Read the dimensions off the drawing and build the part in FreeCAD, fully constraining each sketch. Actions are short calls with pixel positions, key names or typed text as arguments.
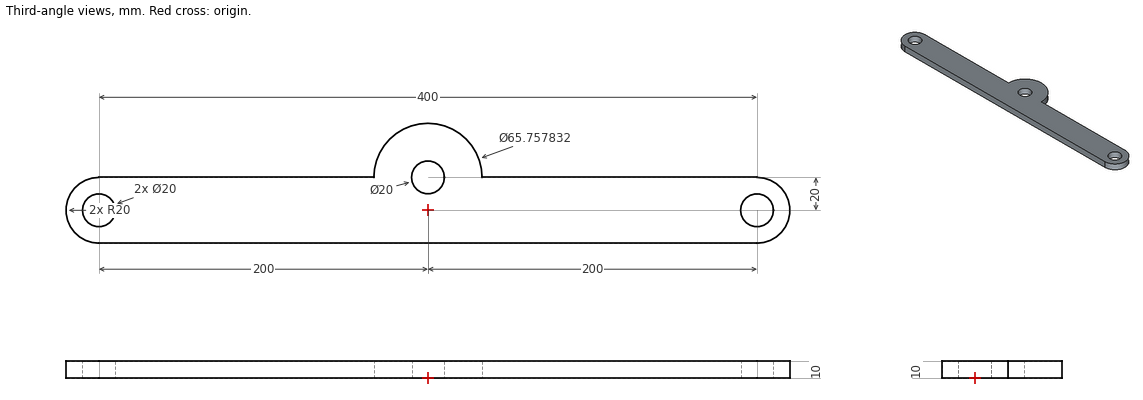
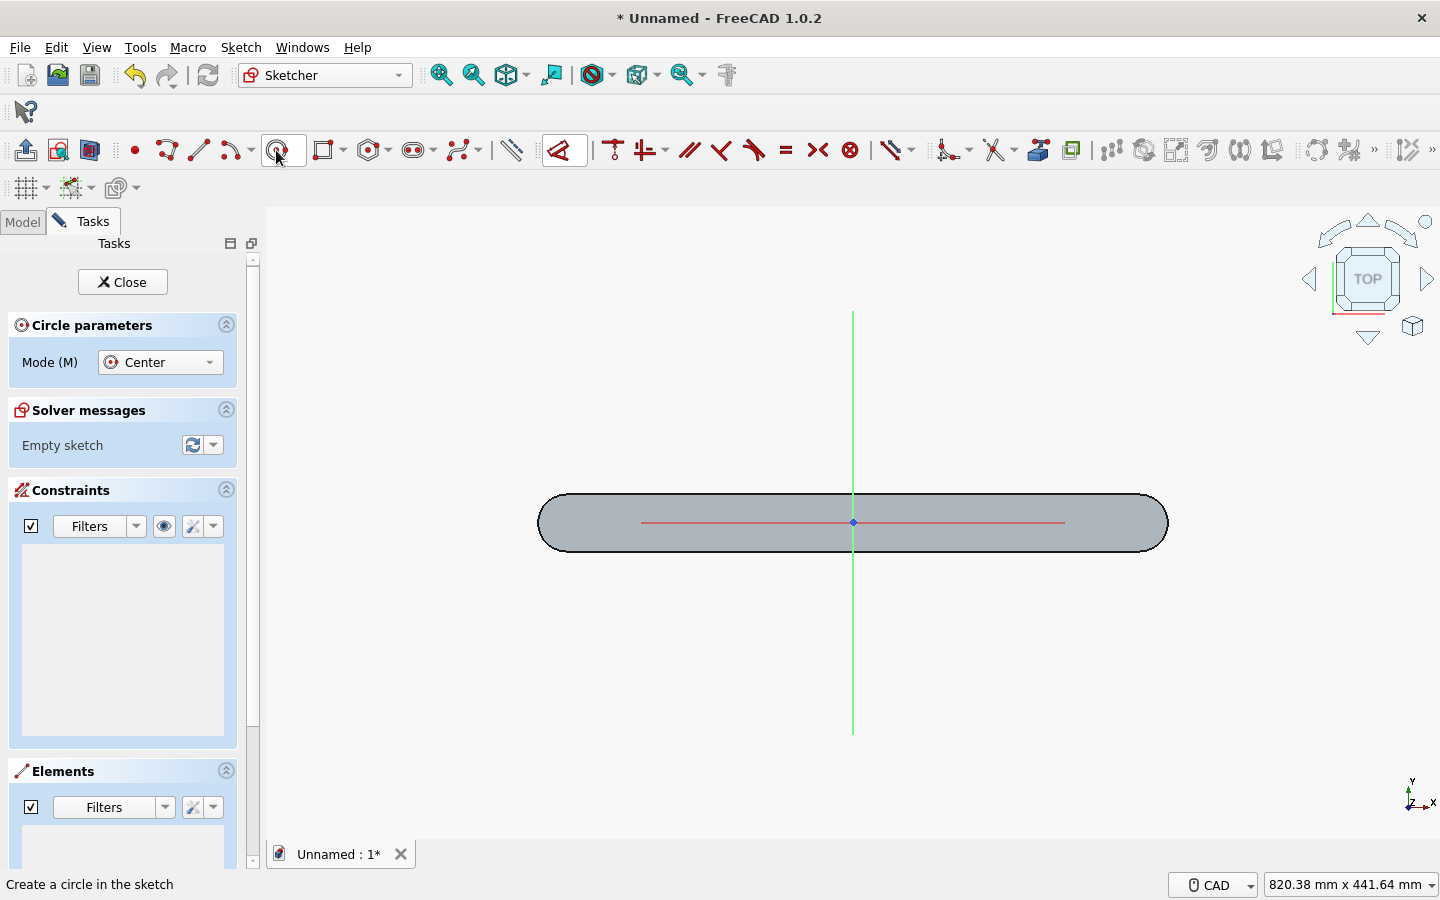
scroll(567, 523, up, 3)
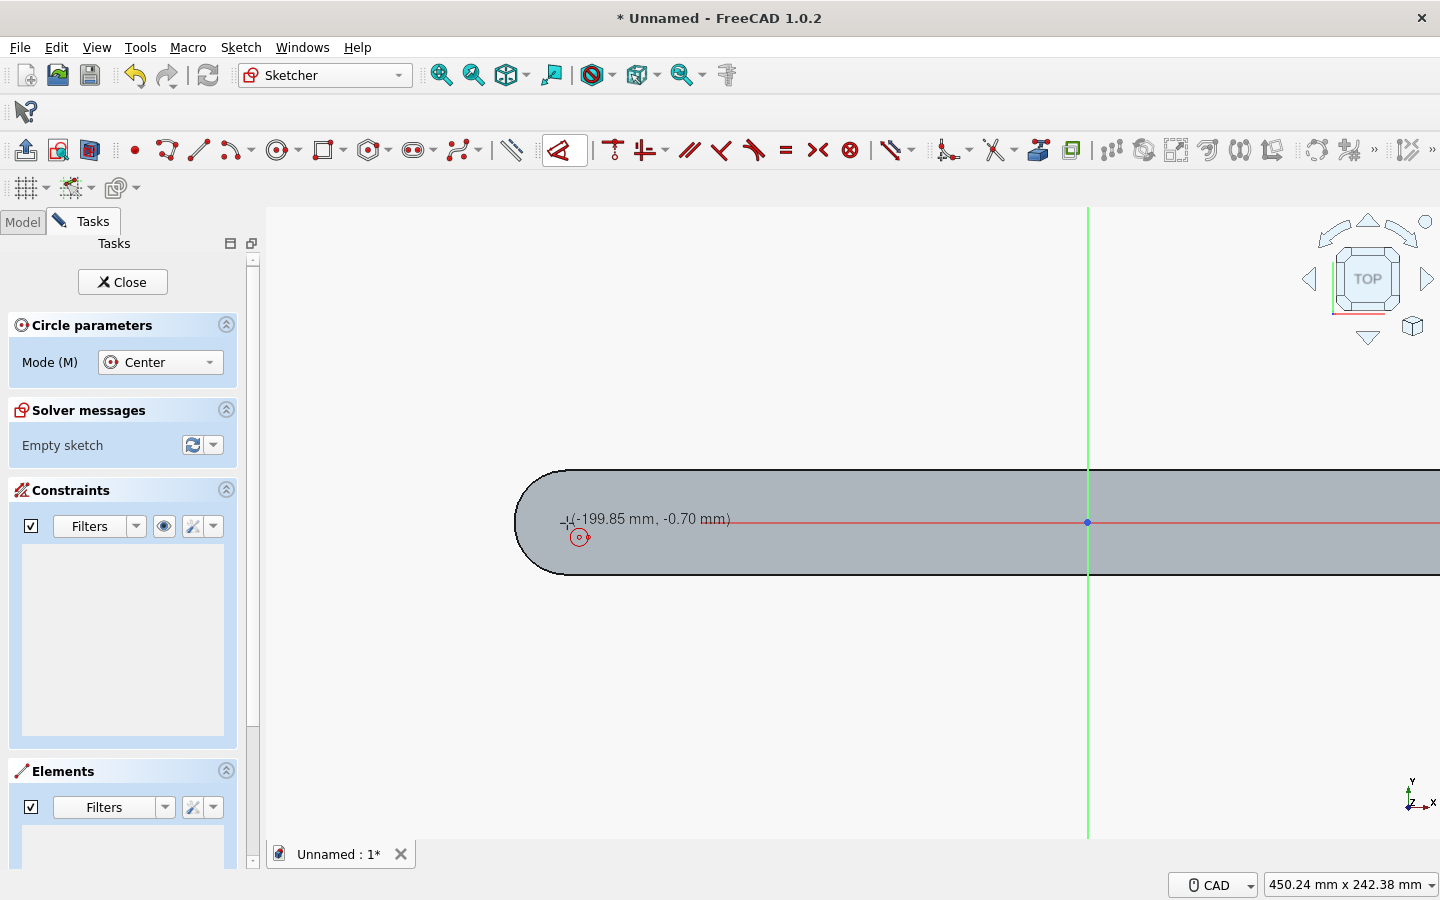
click(566, 523)
move(585, 504)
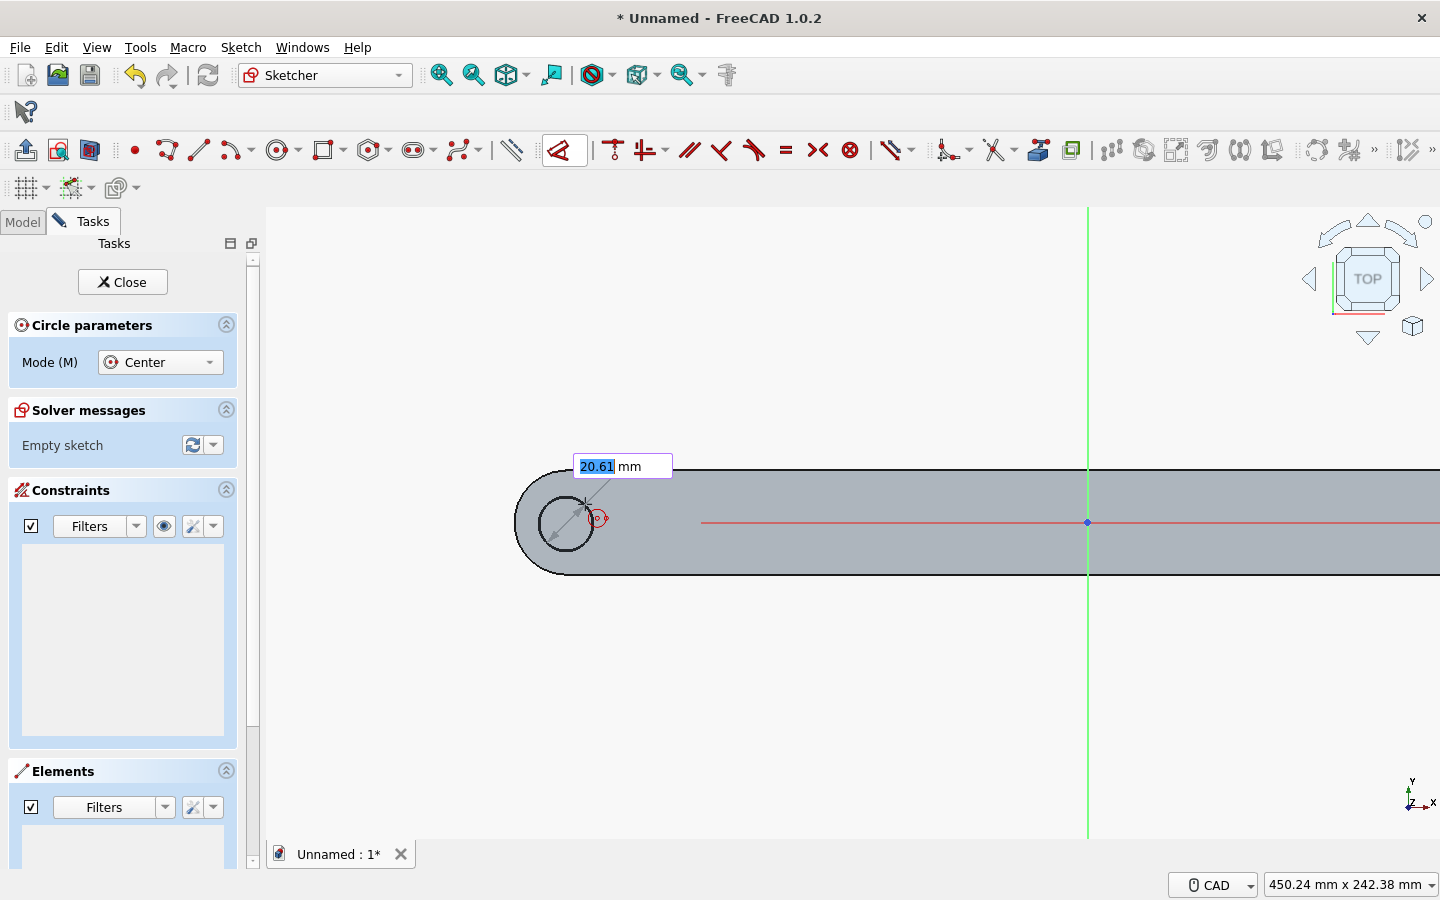
text(20)
key(Return)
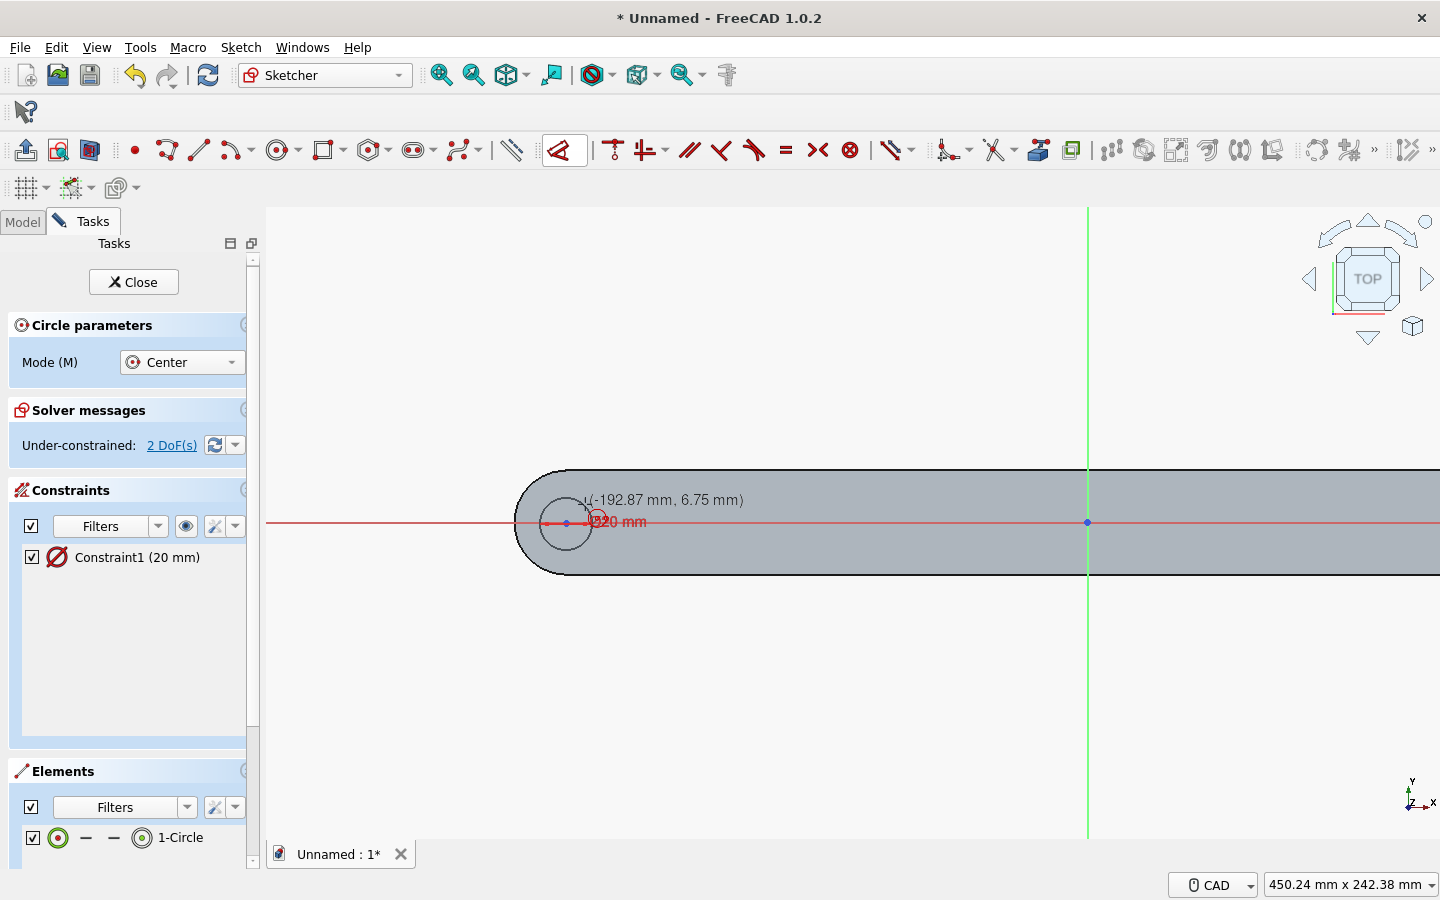
scroll(294, 524, down, 2)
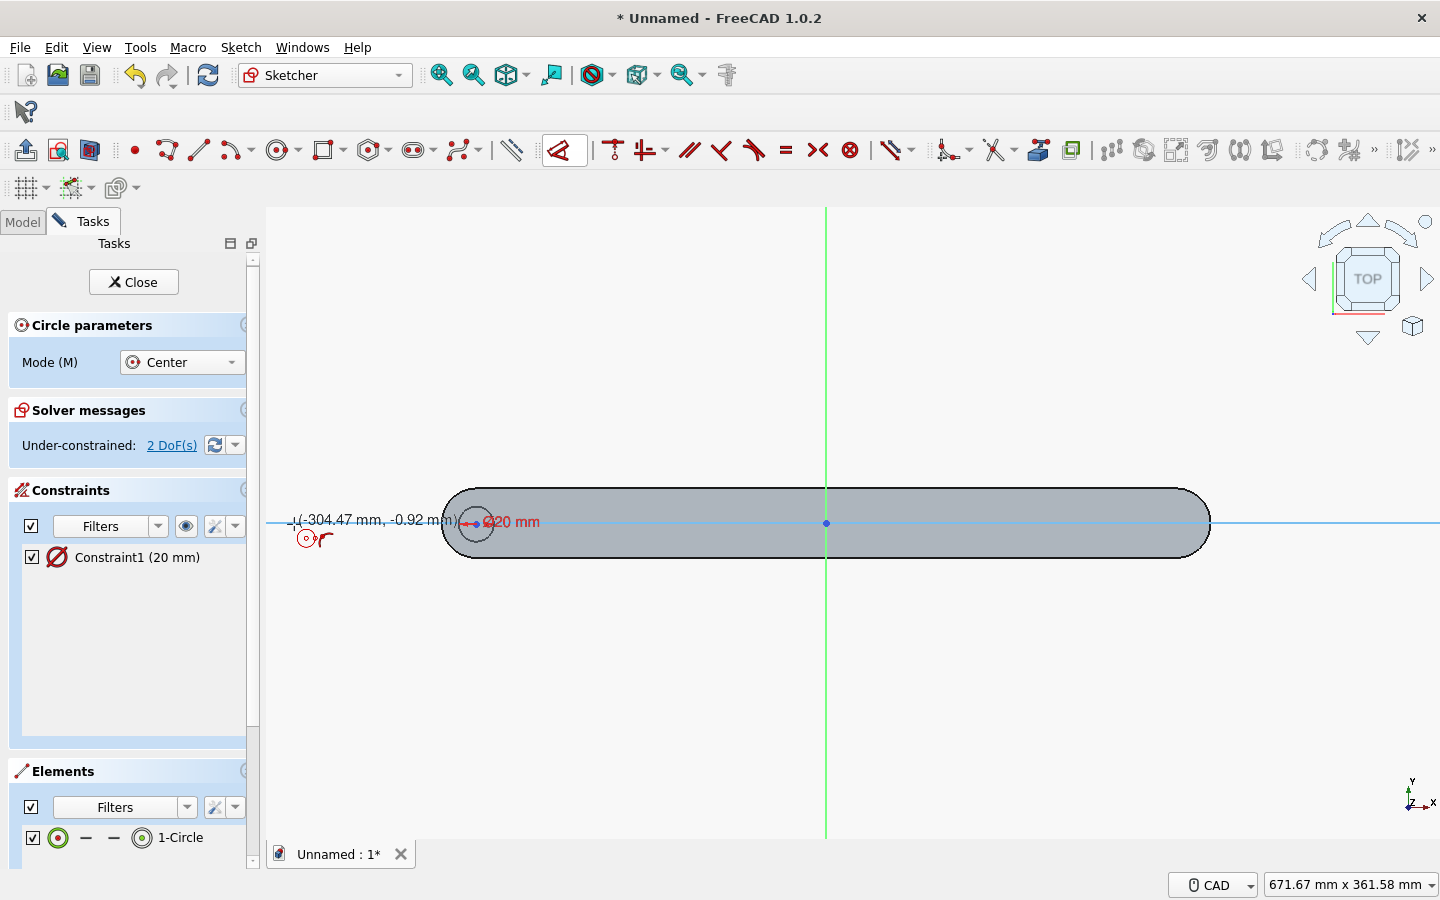
scroll(1176, 523, up, 2)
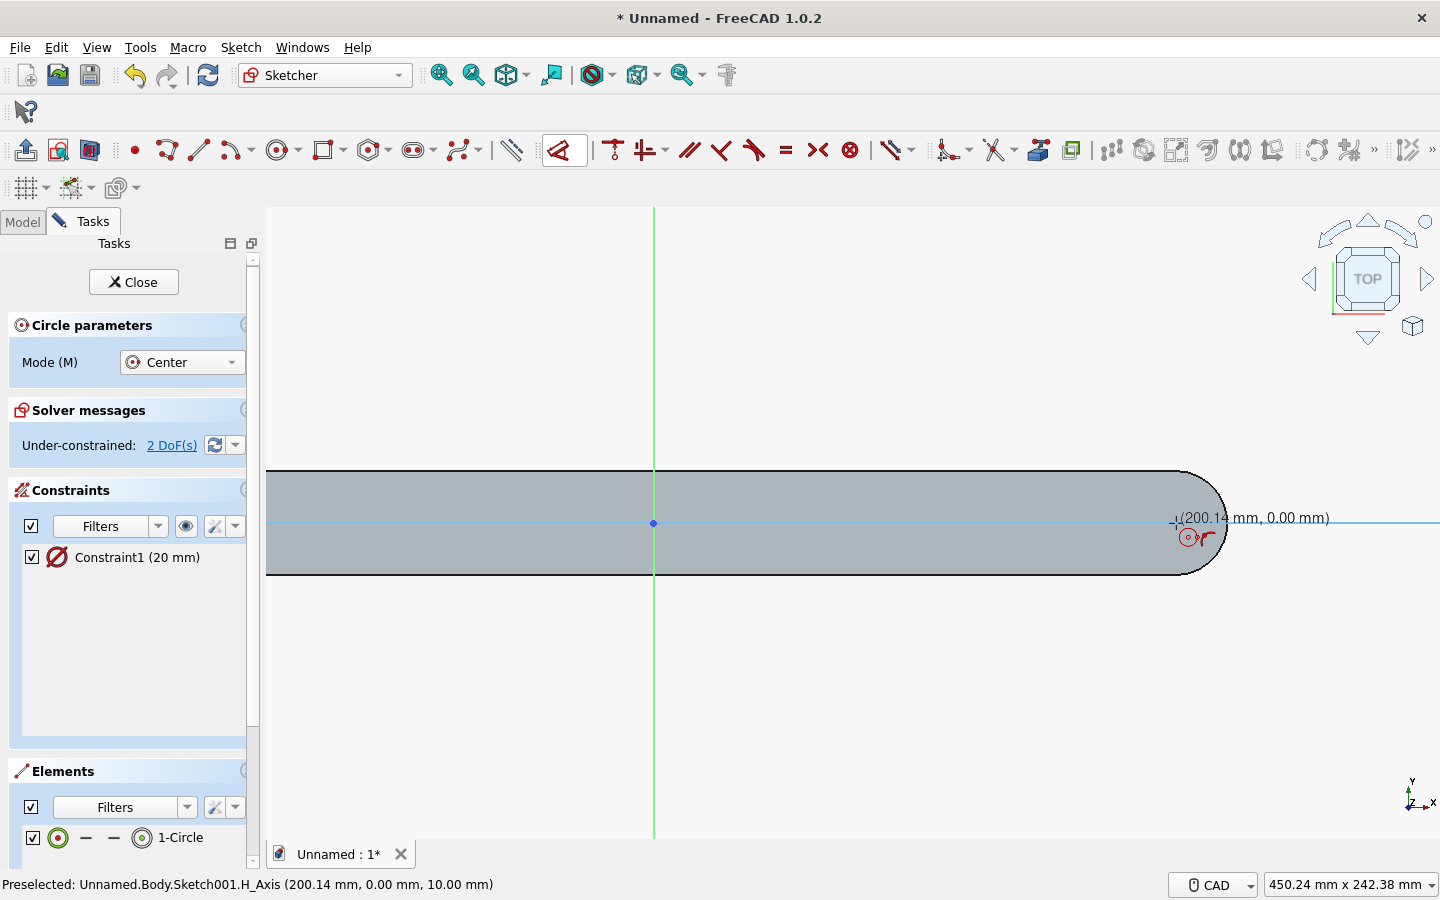
click(1175, 523)
move(1194, 505)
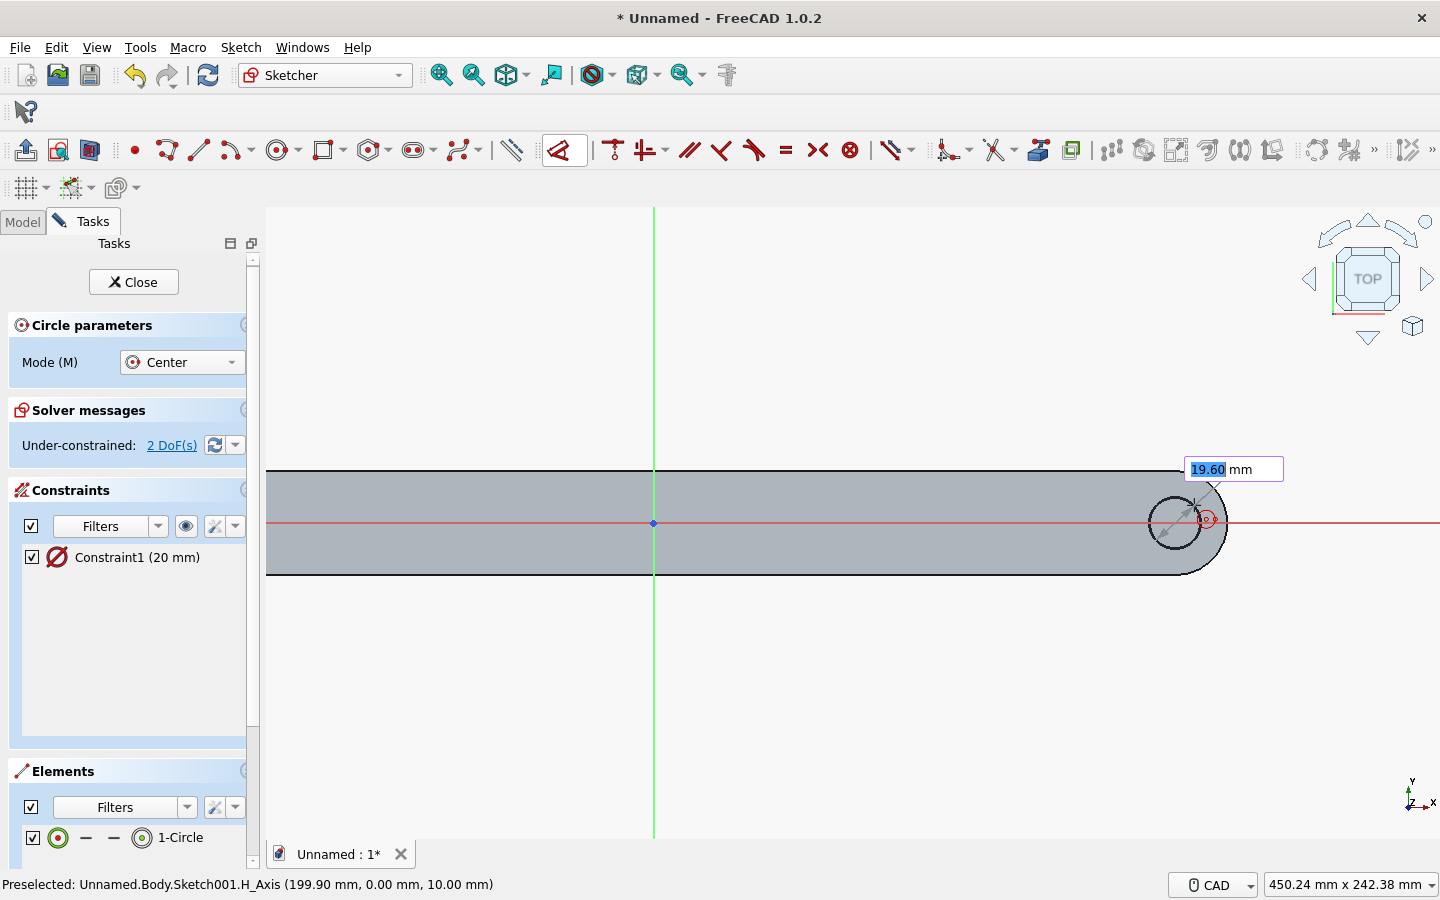
text(20)
key(Return)
key(Escape)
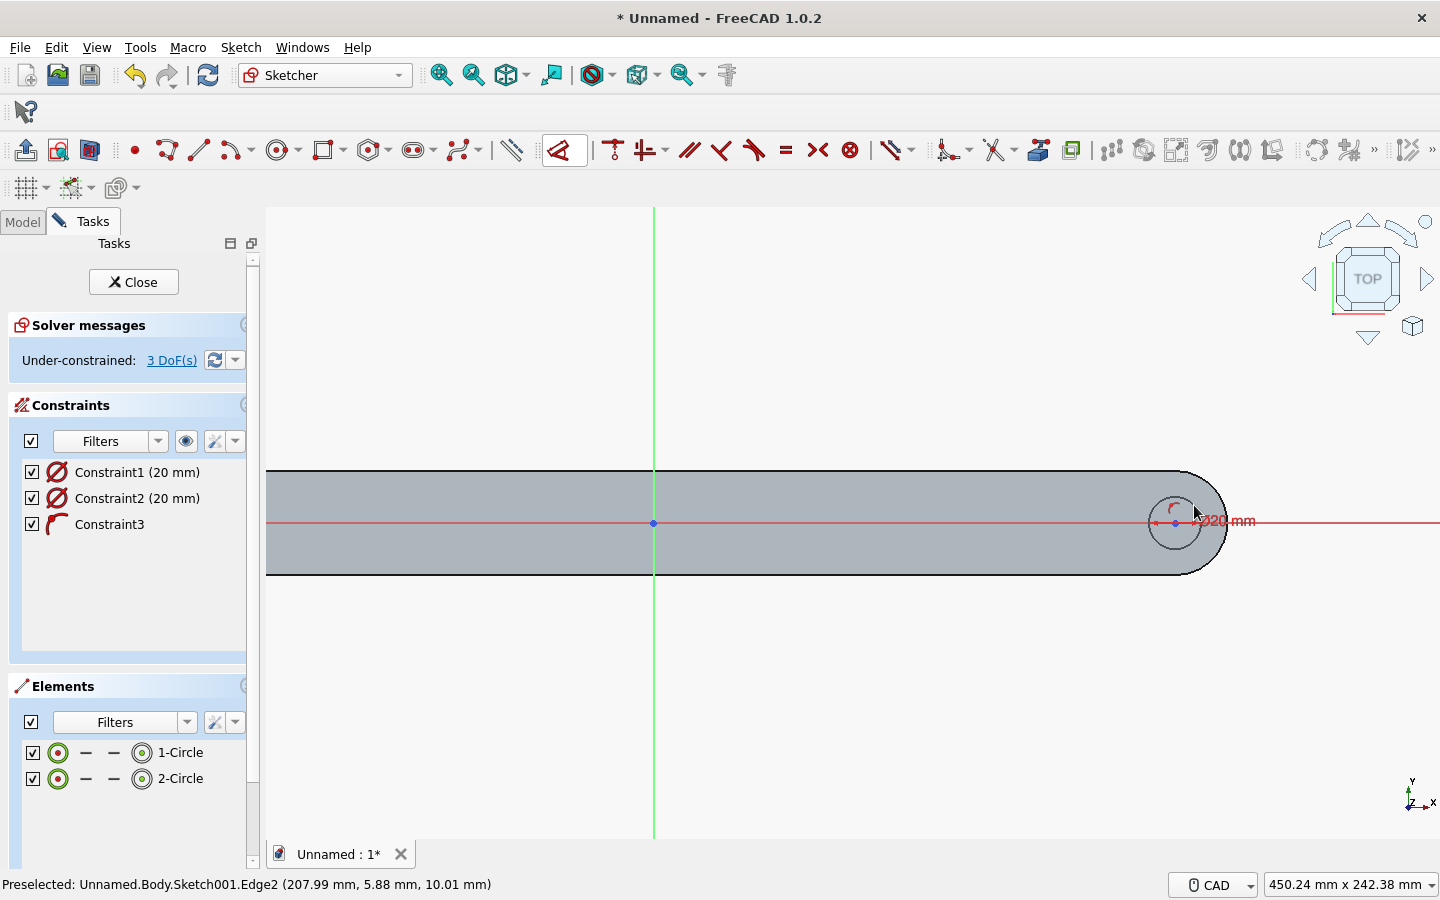
scroll(1050, 523, down, 2)